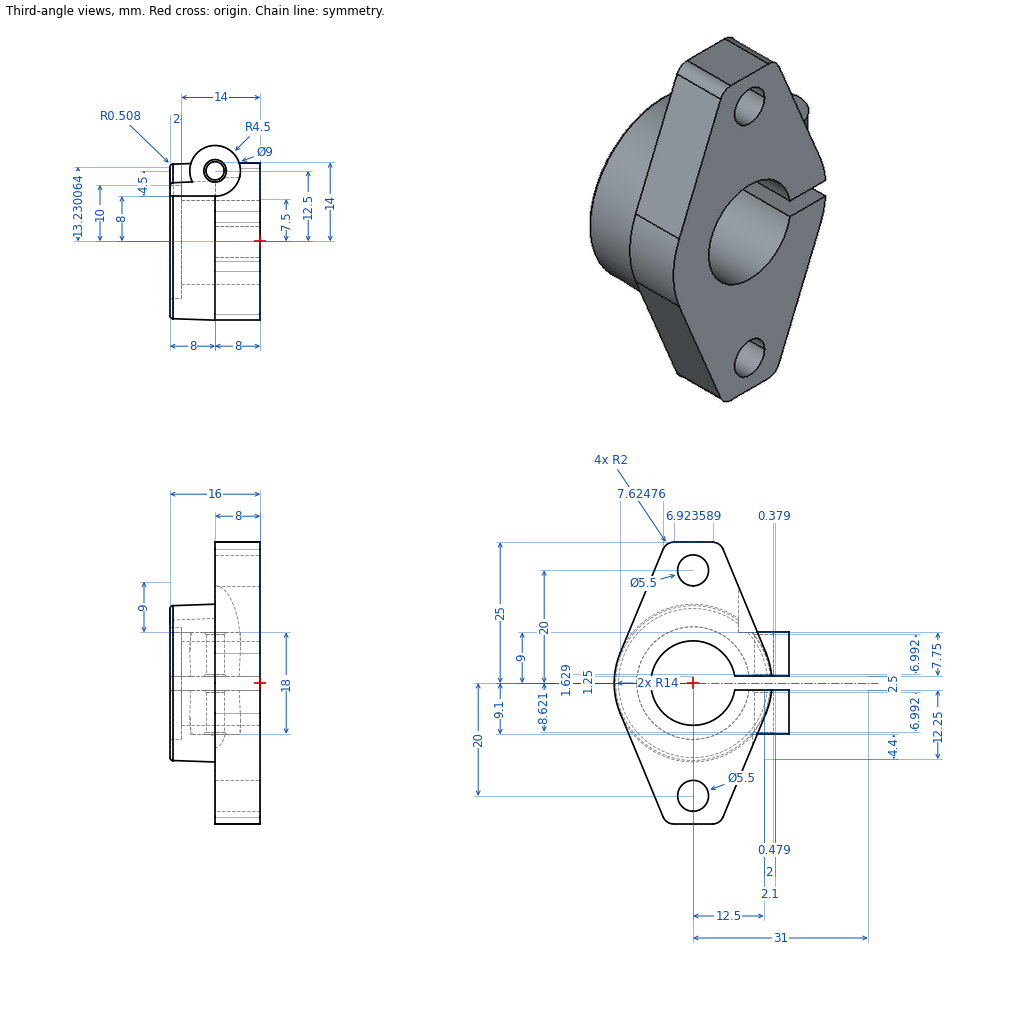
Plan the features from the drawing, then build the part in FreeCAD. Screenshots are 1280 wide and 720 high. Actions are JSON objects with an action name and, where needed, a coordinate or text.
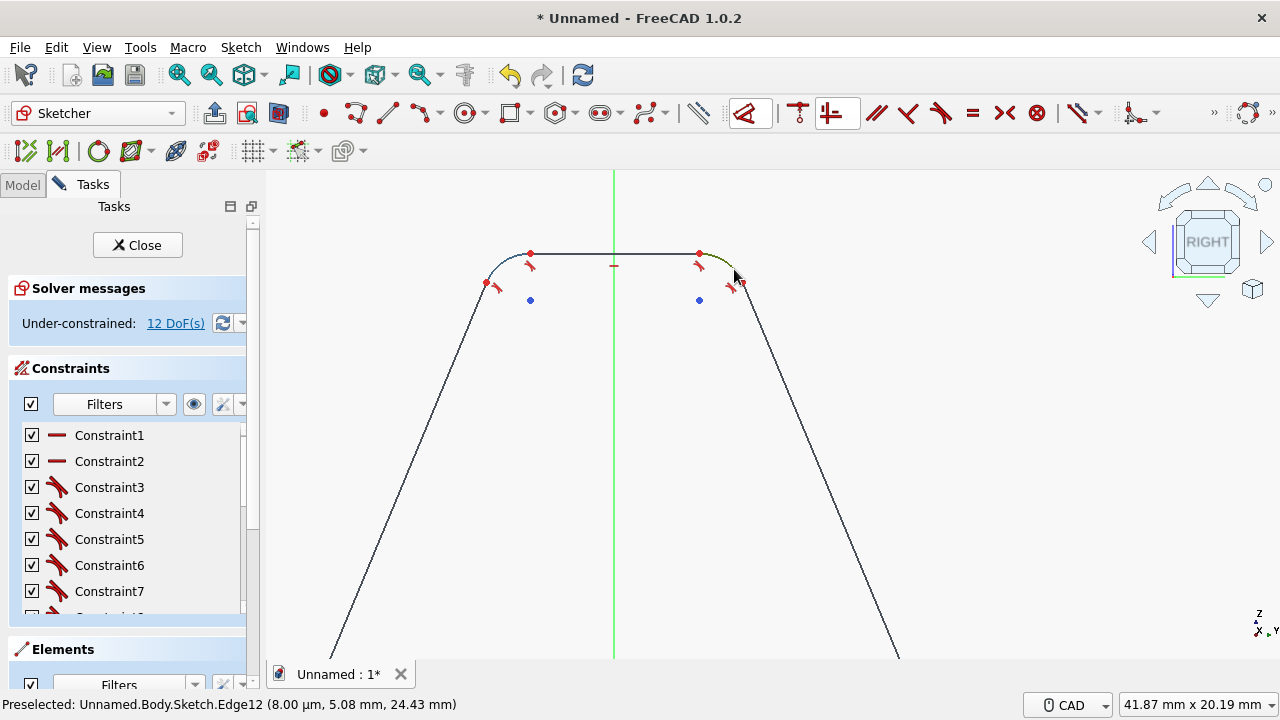
{"action": "left_click", "coordinate": [974, 114]}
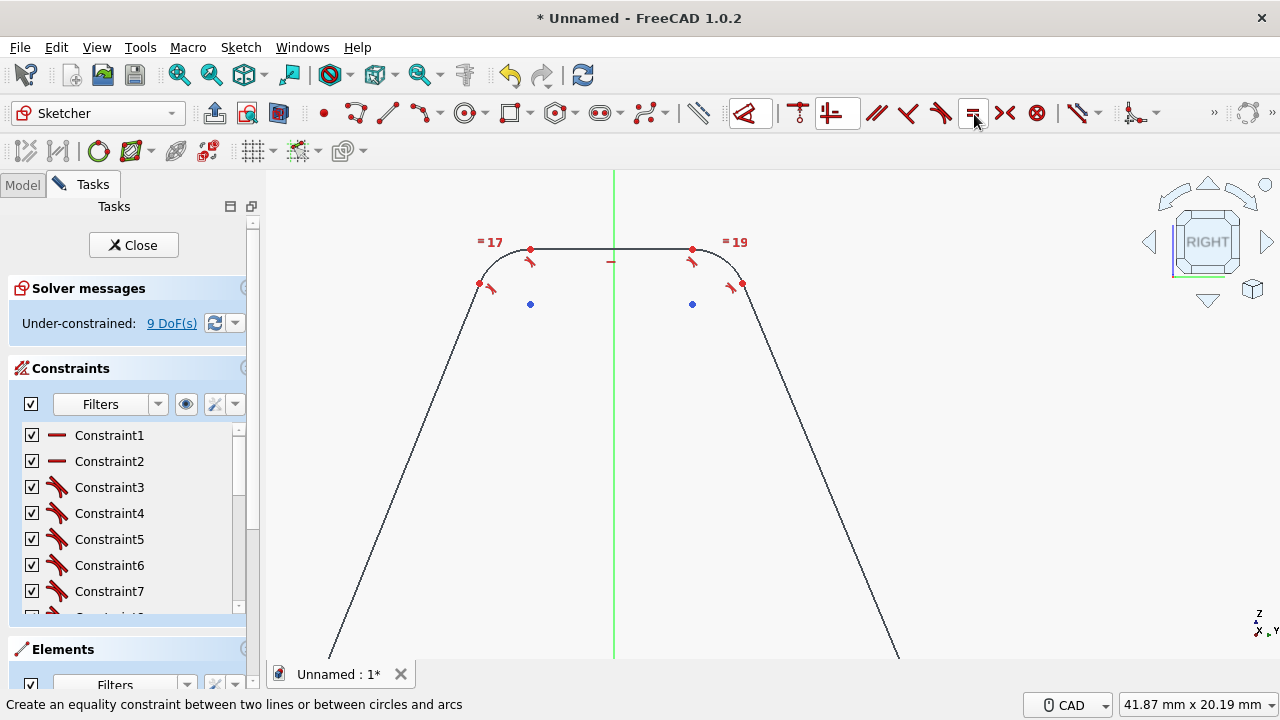
{"action": "scroll", "coordinate": [734, 267], "scroll_direction": "down", "scroll_amount": 7}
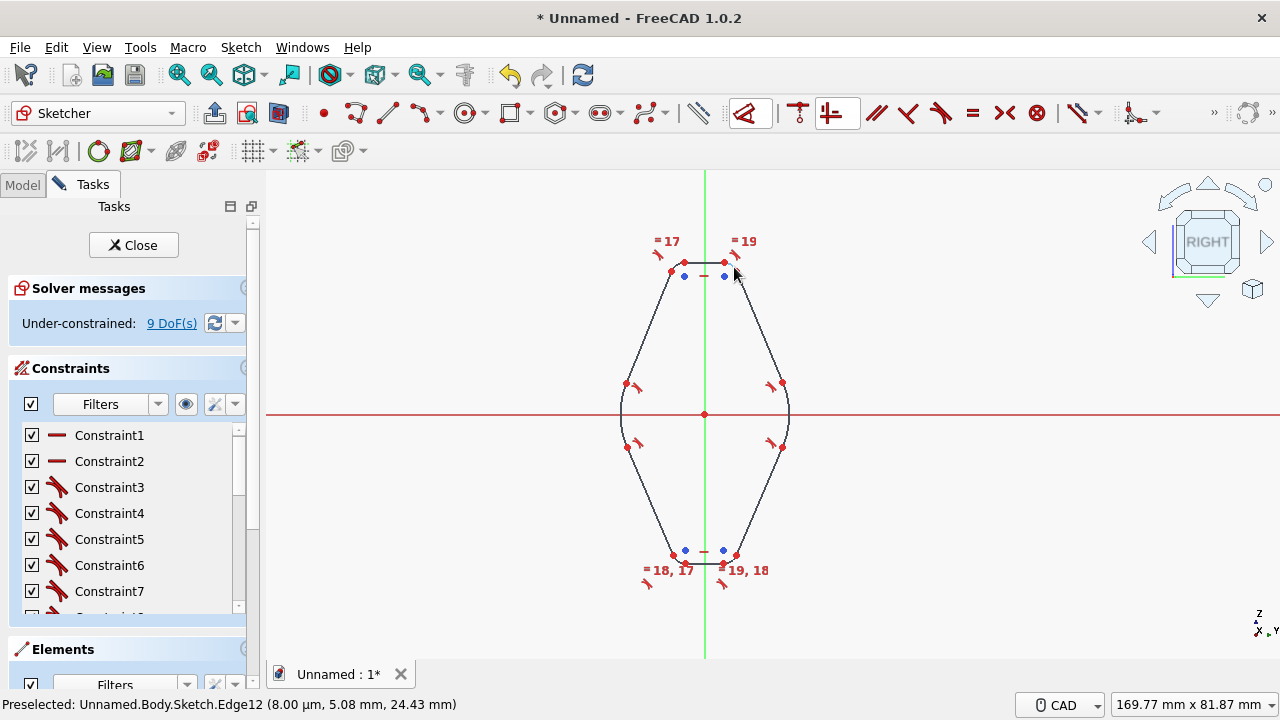
{"action": "left_click", "coordinate": [621, 402]}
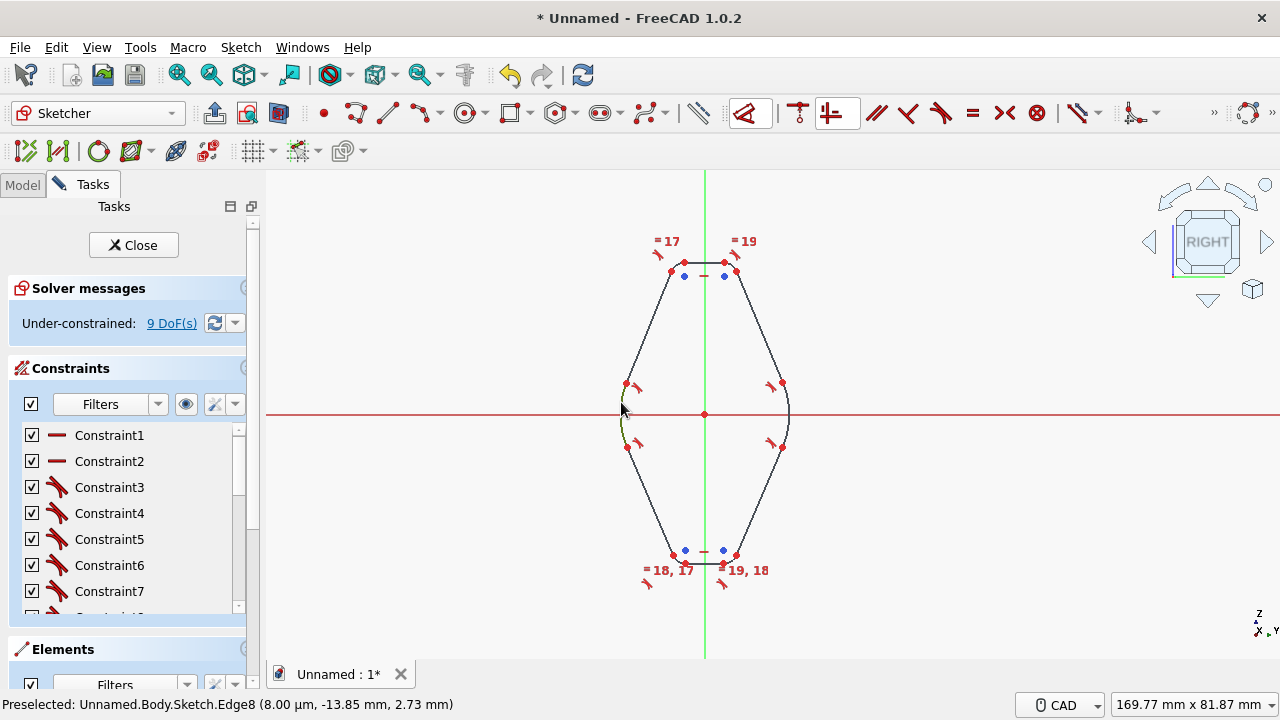
{"action": "left_click", "coordinate": [788, 428]}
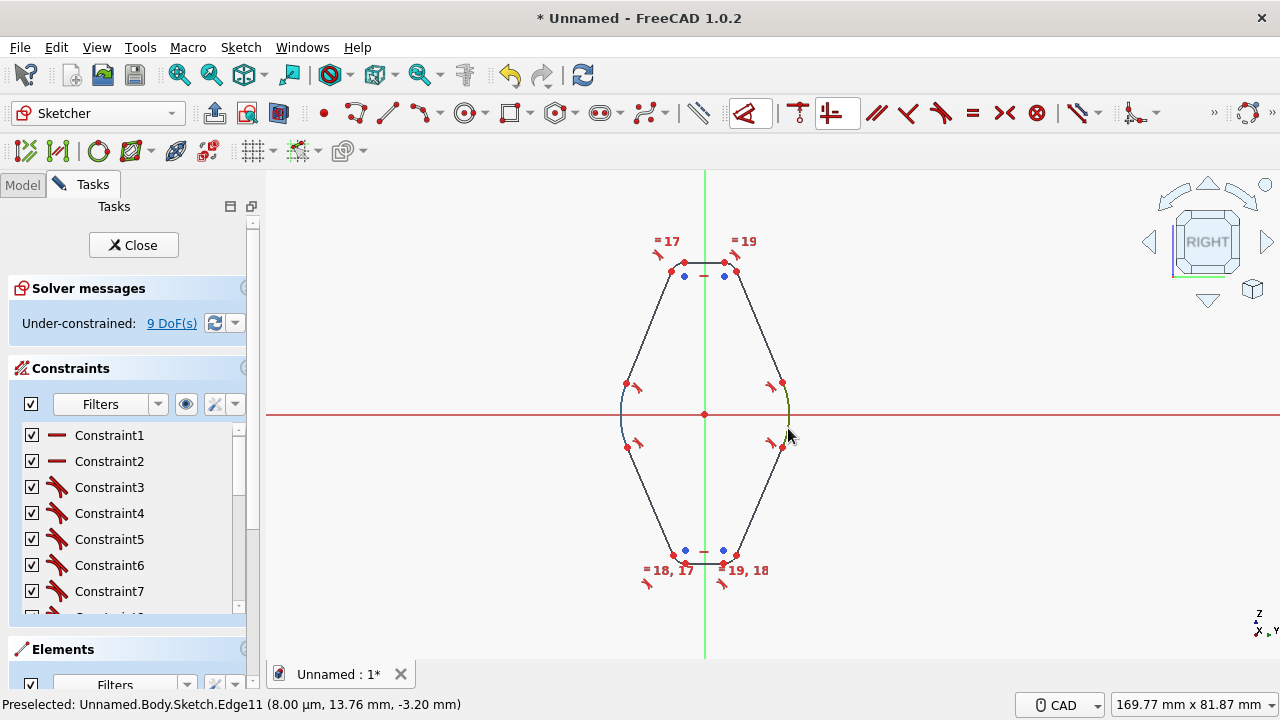
{"action": "key", "text": "e"}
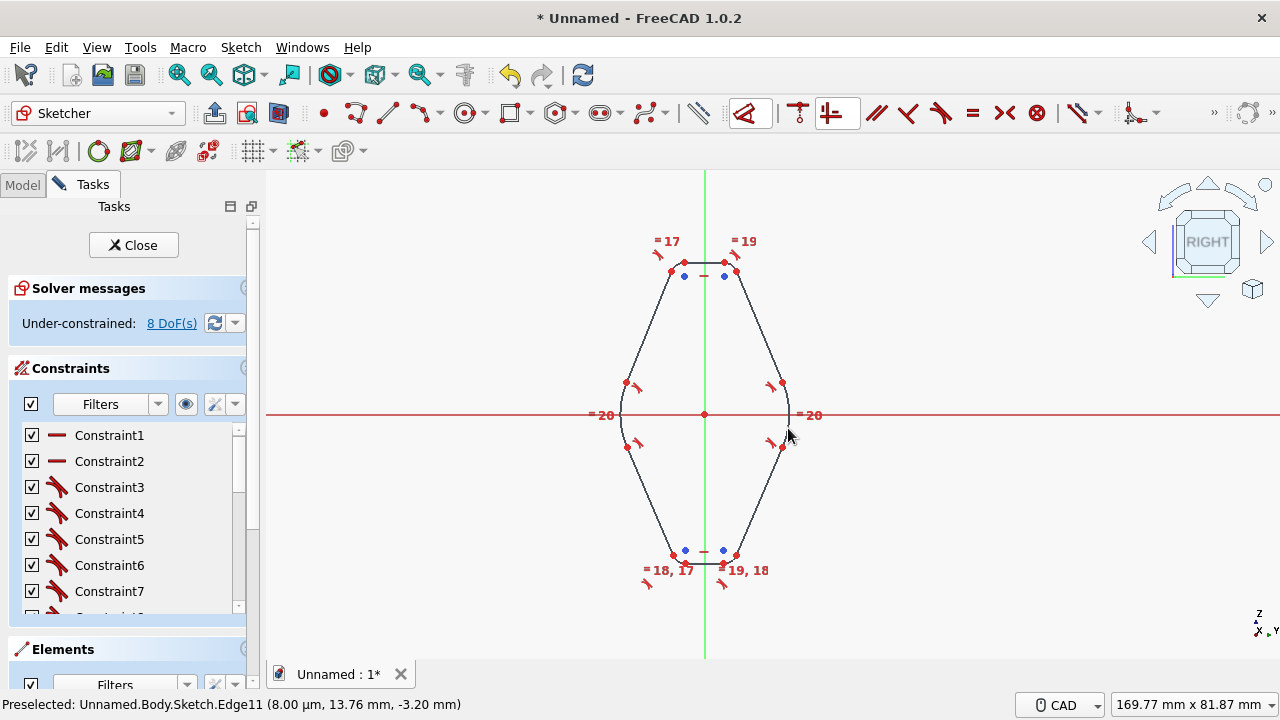
{"action": "left_click", "coordinate": [684, 276]}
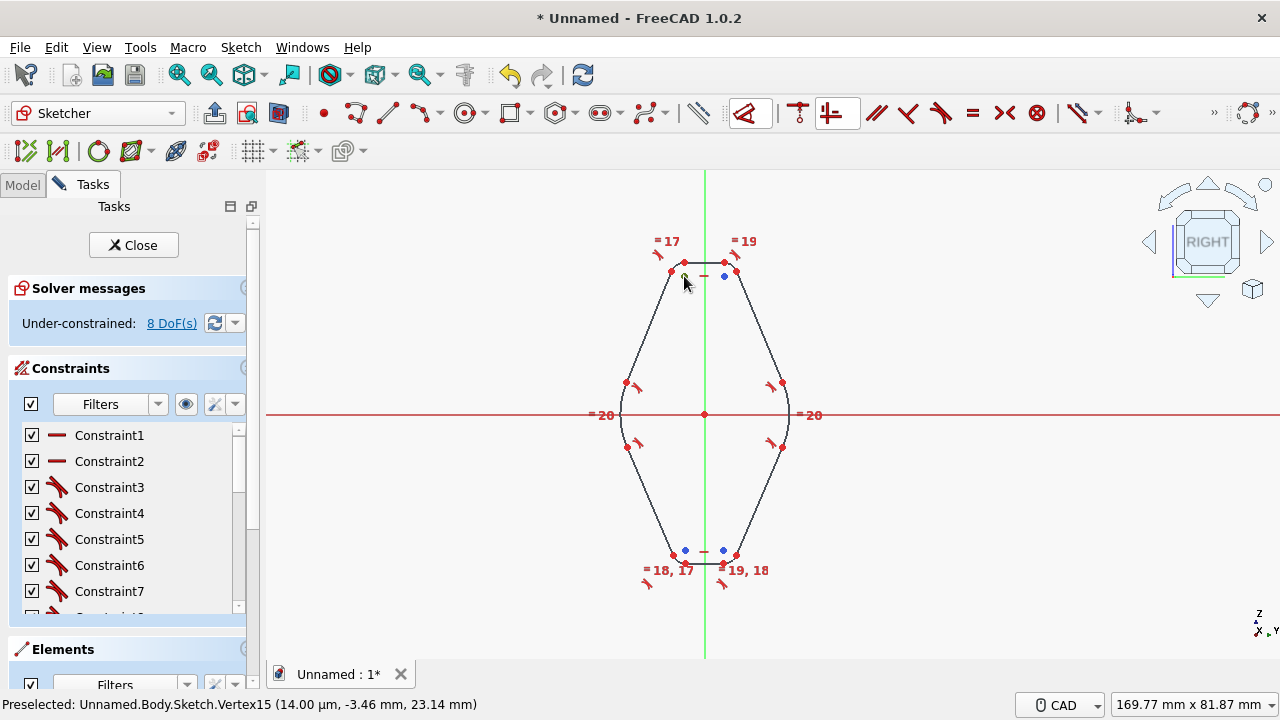
{"action": "left_click", "coordinate": [686, 550]}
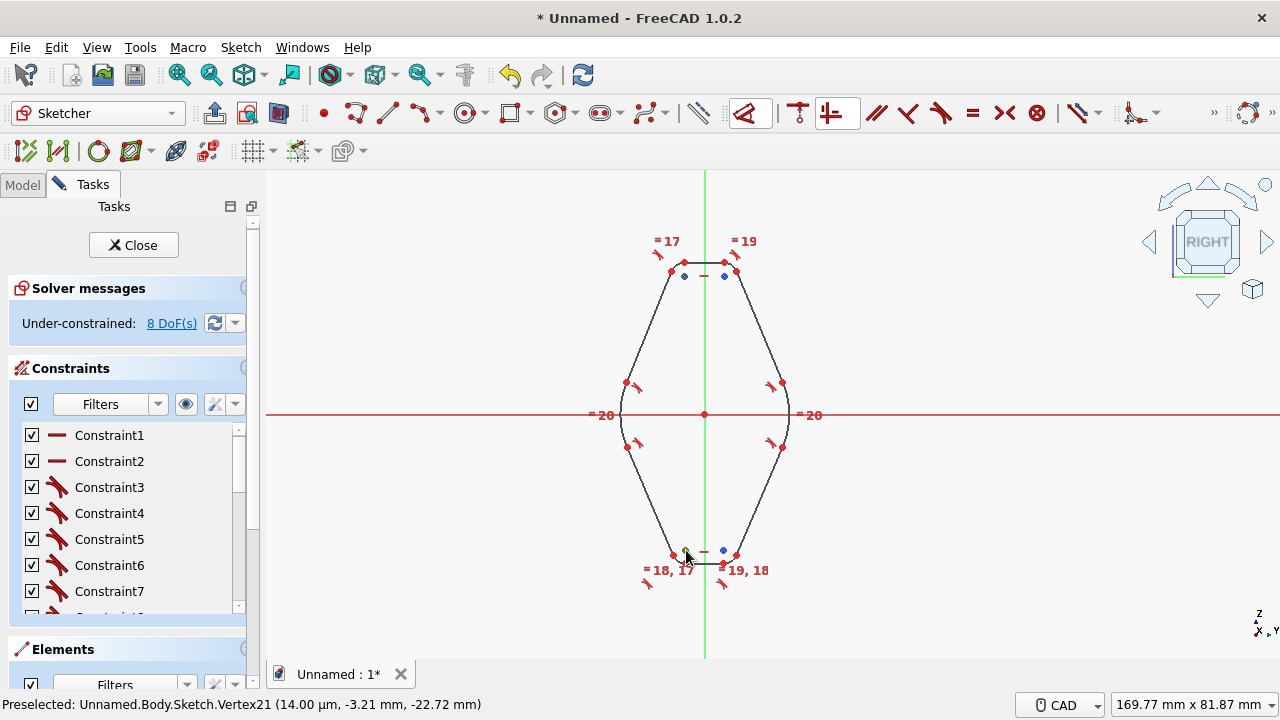
{"action": "left_click", "coordinate": [353, 415]}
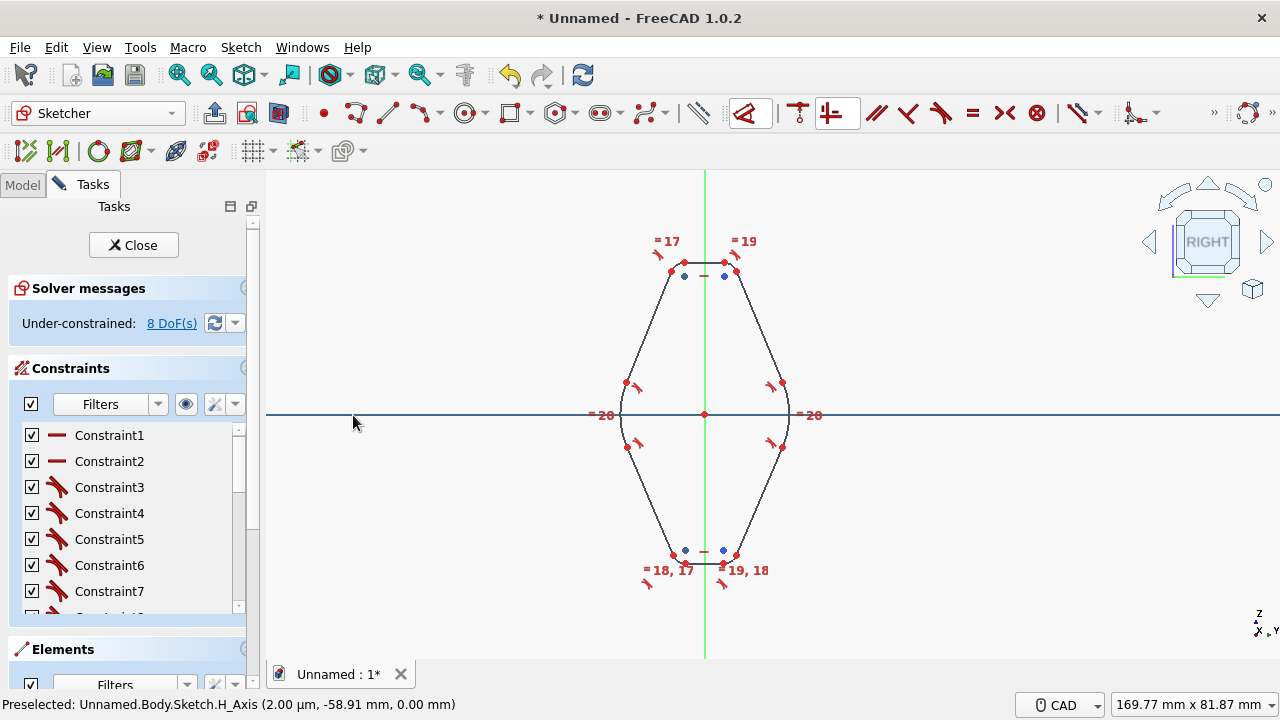
{"action": "left_click", "coordinate": [1006, 114]}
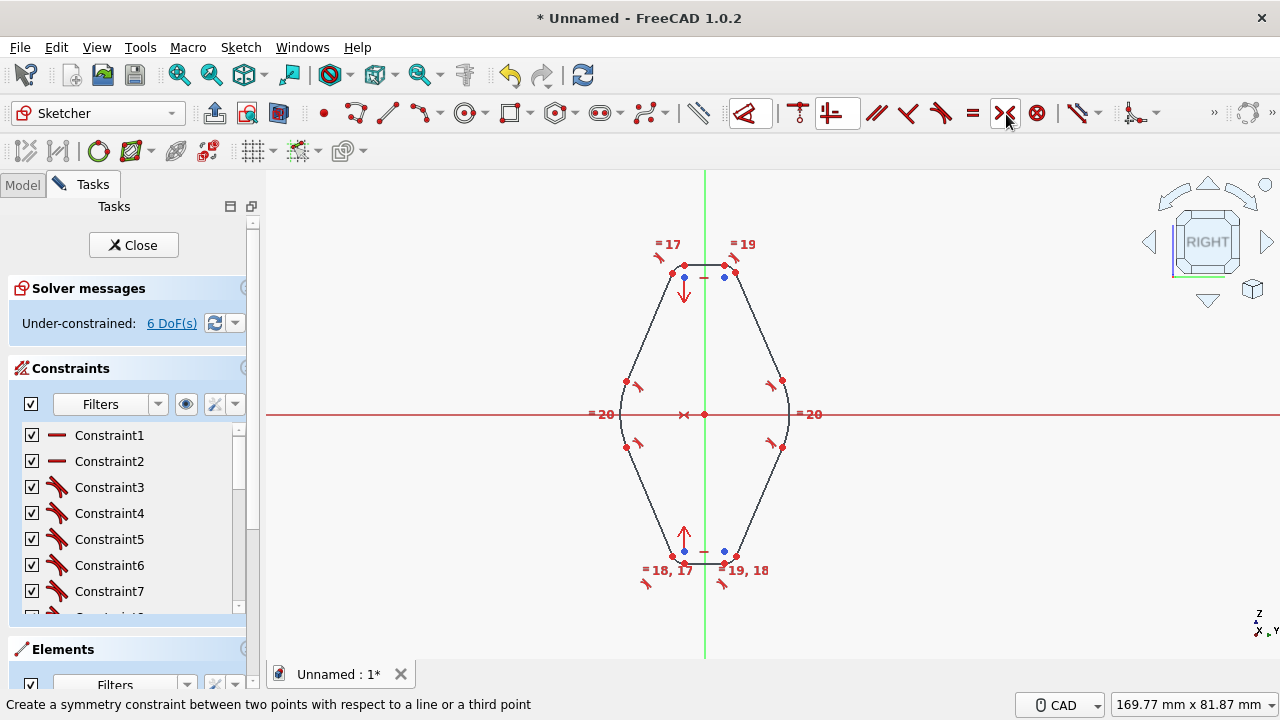
{"action": "scroll", "coordinate": [677, 267], "scroll_direction": "up", "scroll_amount": 7}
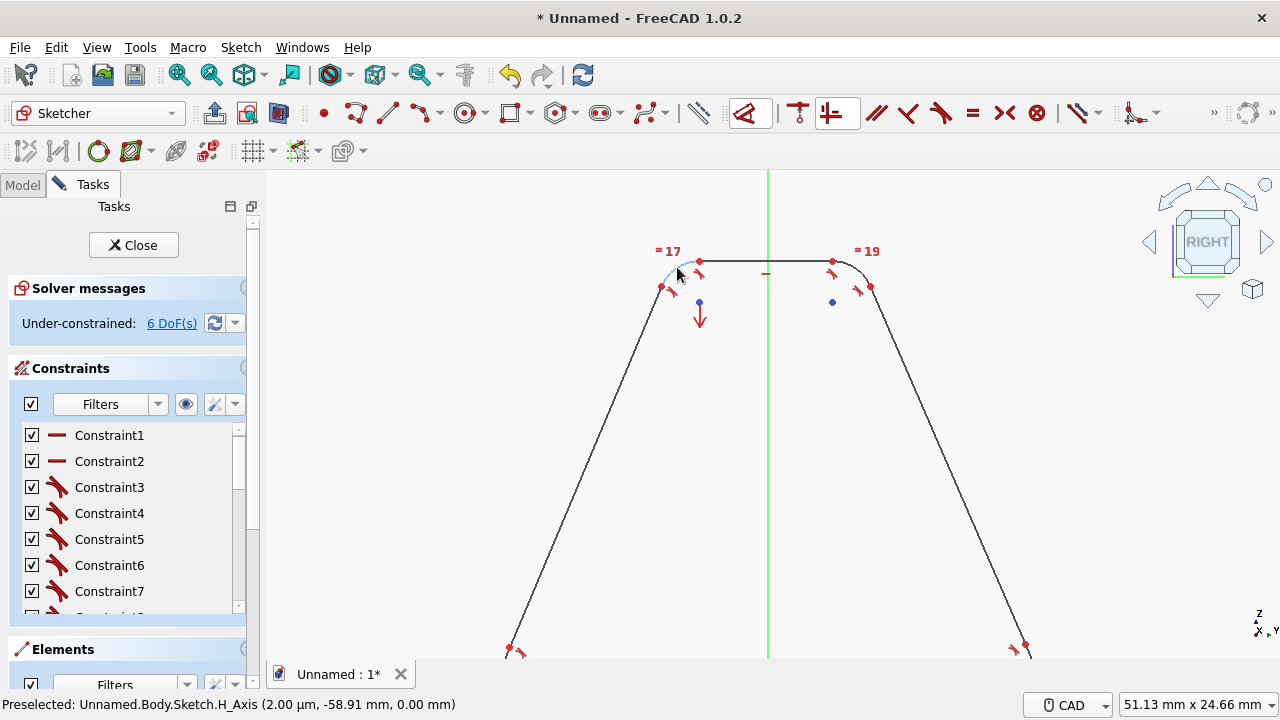
{"action": "left_click", "coordinate": [677, 268]}